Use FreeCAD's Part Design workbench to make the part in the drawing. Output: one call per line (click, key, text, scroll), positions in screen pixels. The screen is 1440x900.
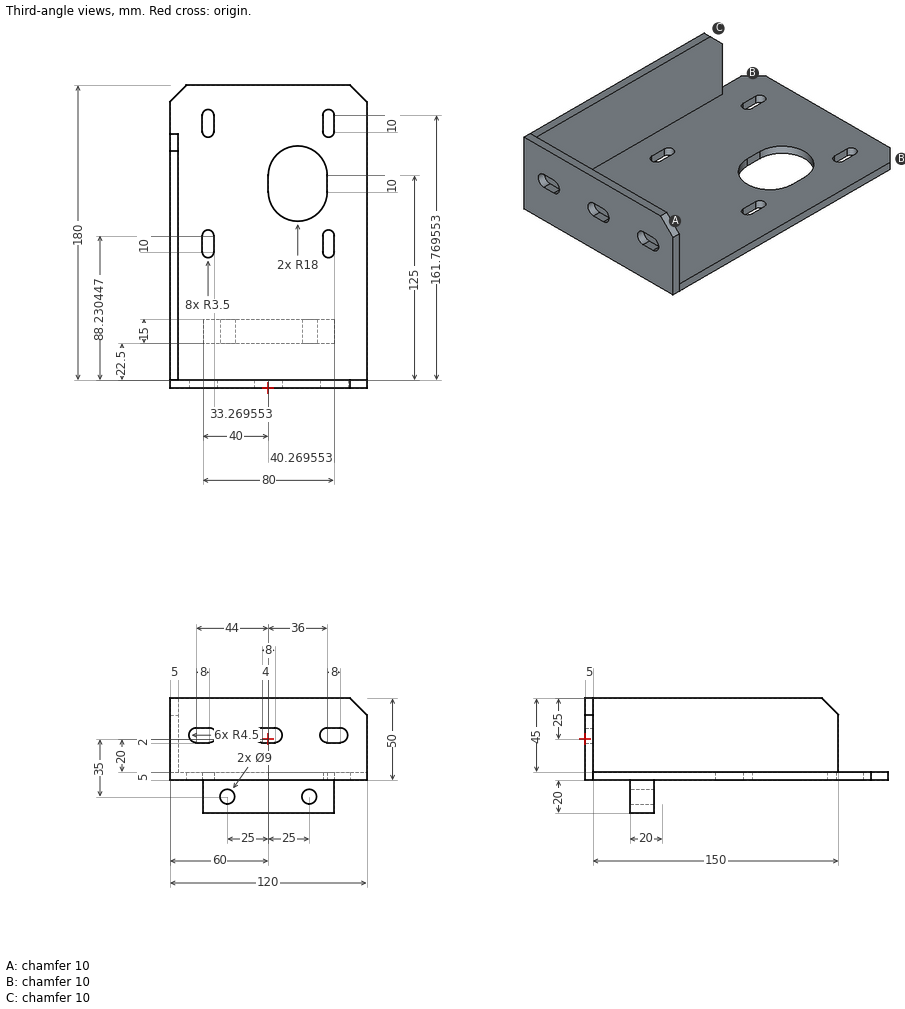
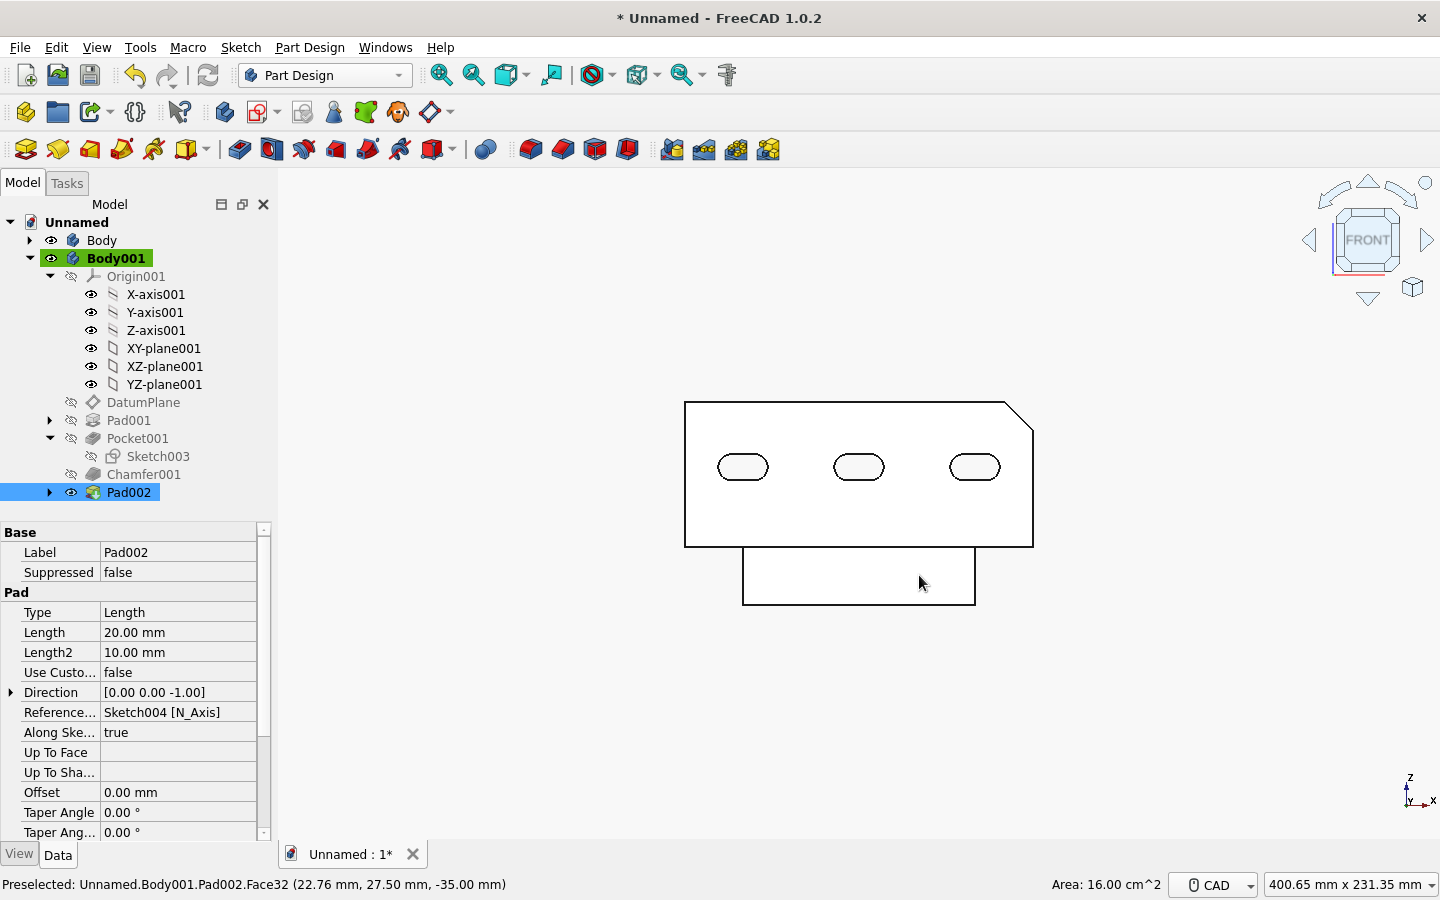
click(258, 112)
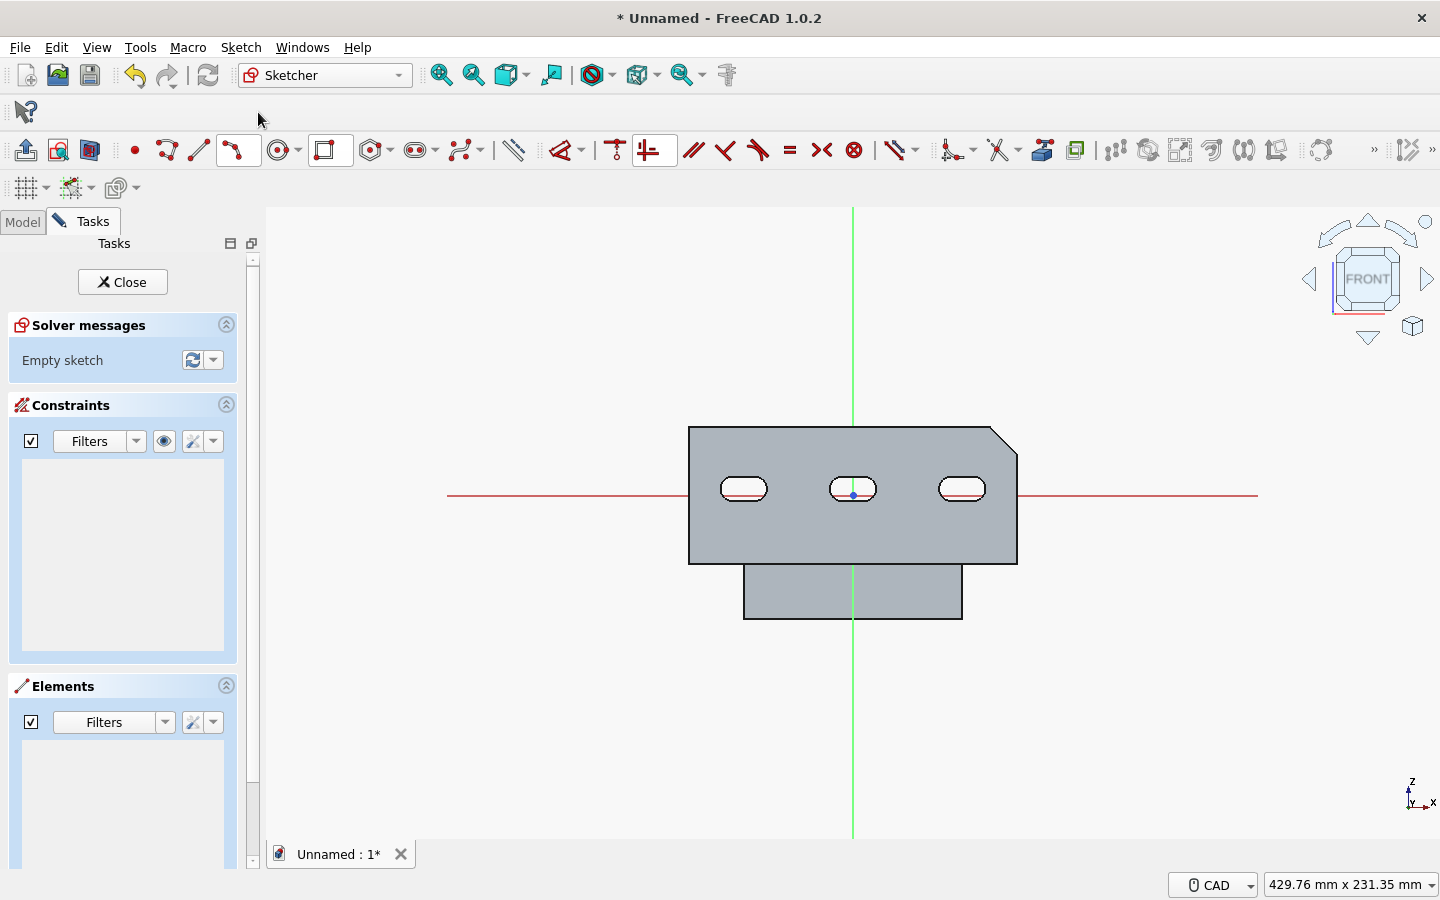
scroll(875, 558, up, 7)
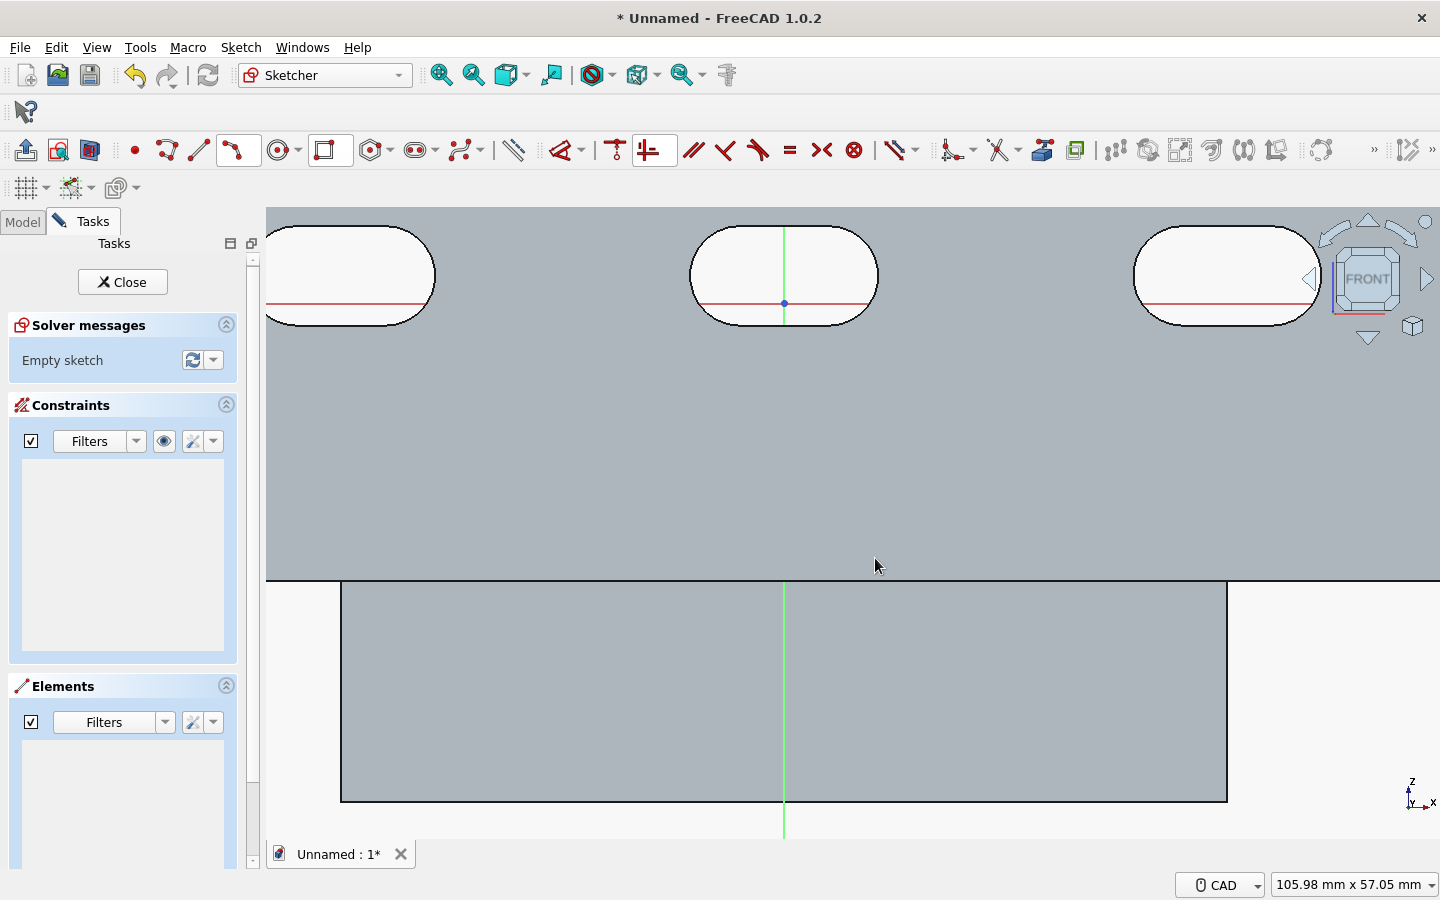
key(g)
key(c)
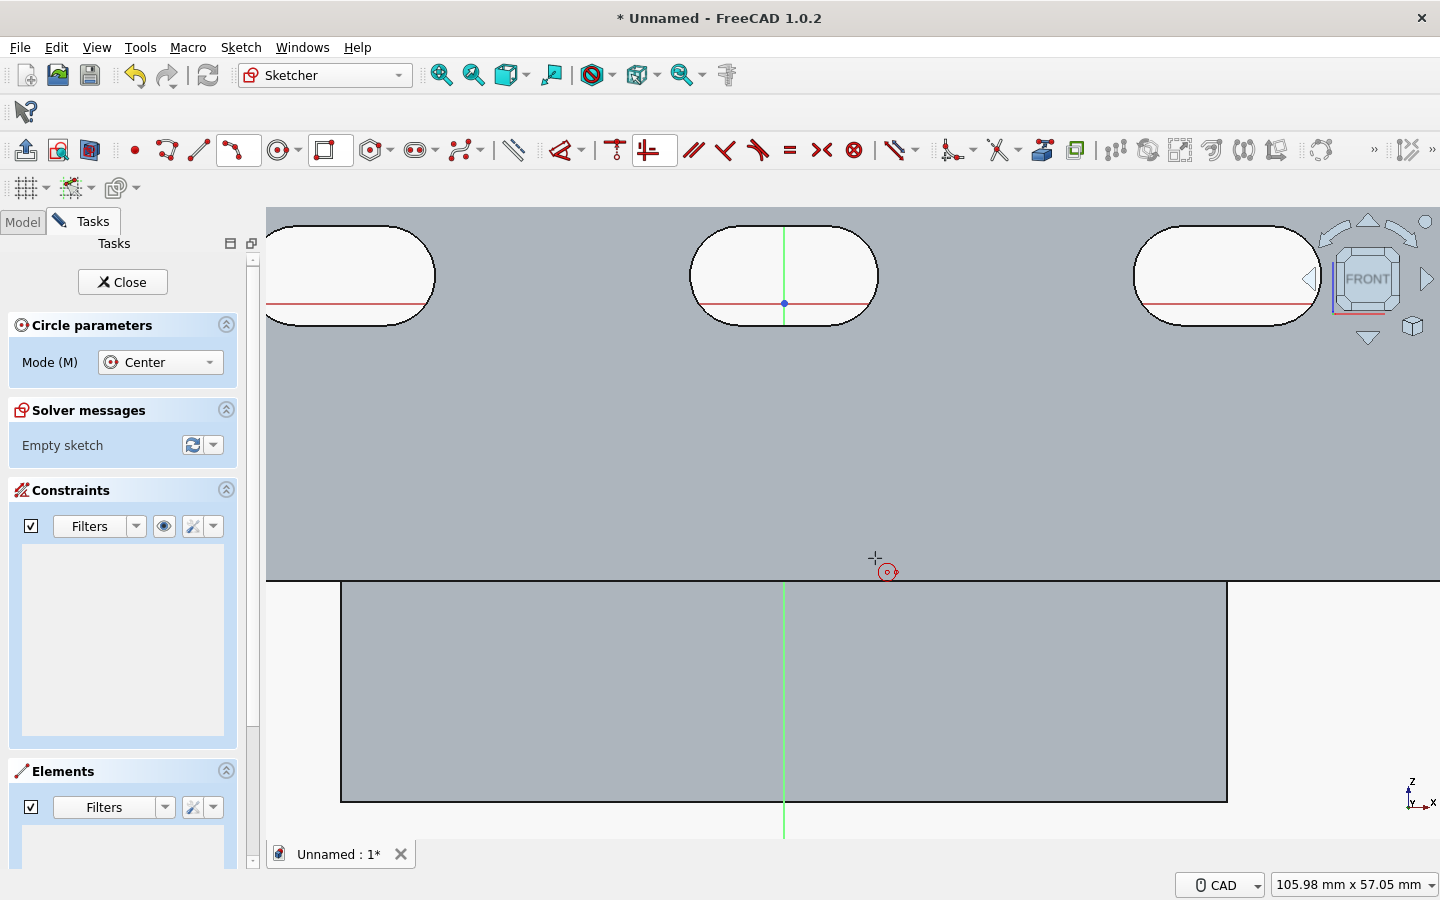
click(507, 691)
click(543, 656)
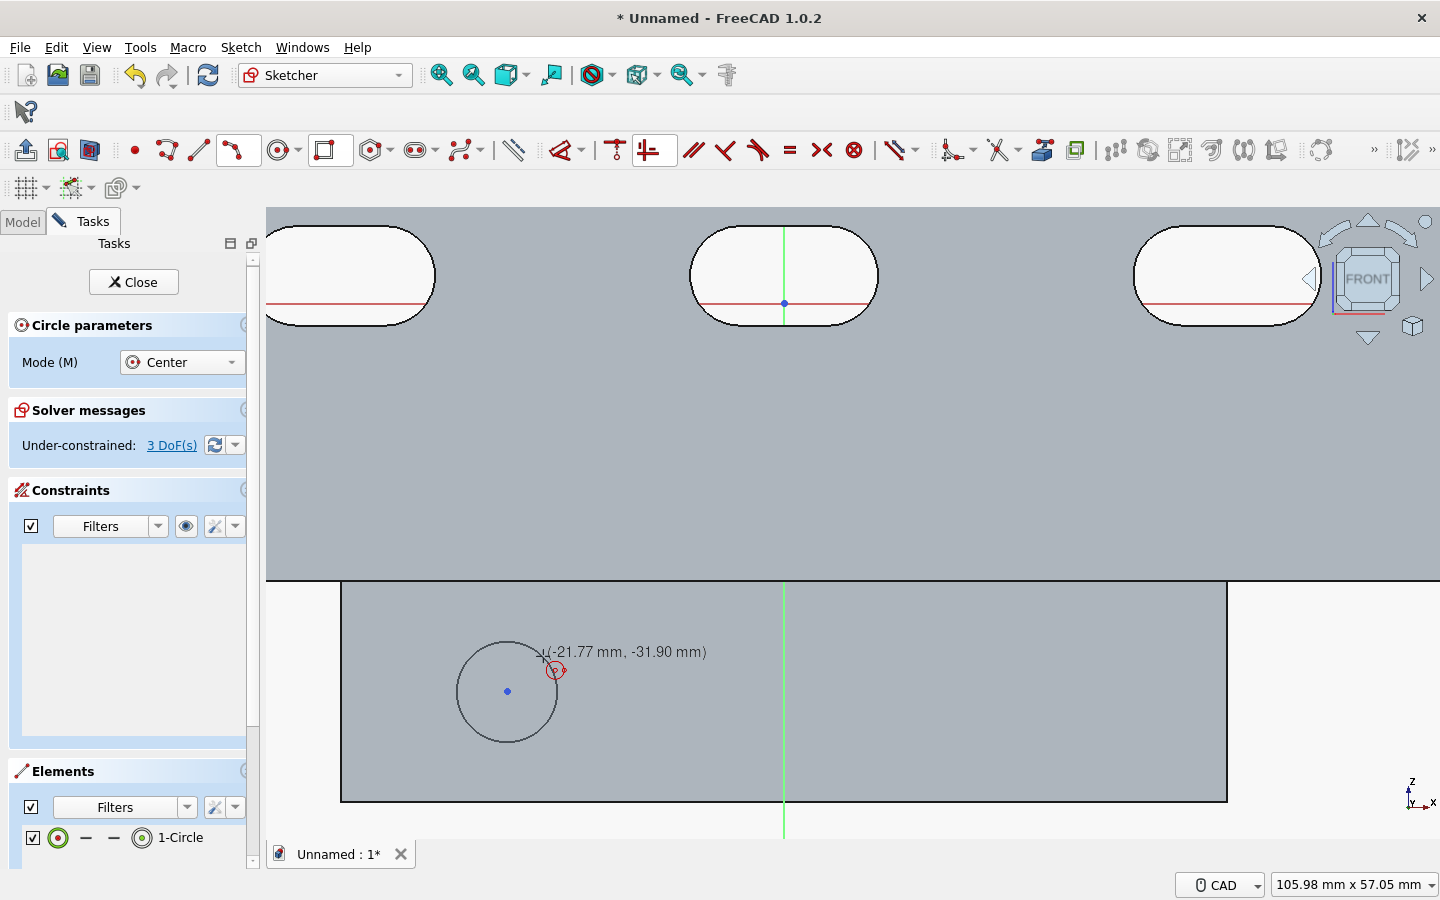
click(1061, 691)
click(1096, 656)
key(Escape)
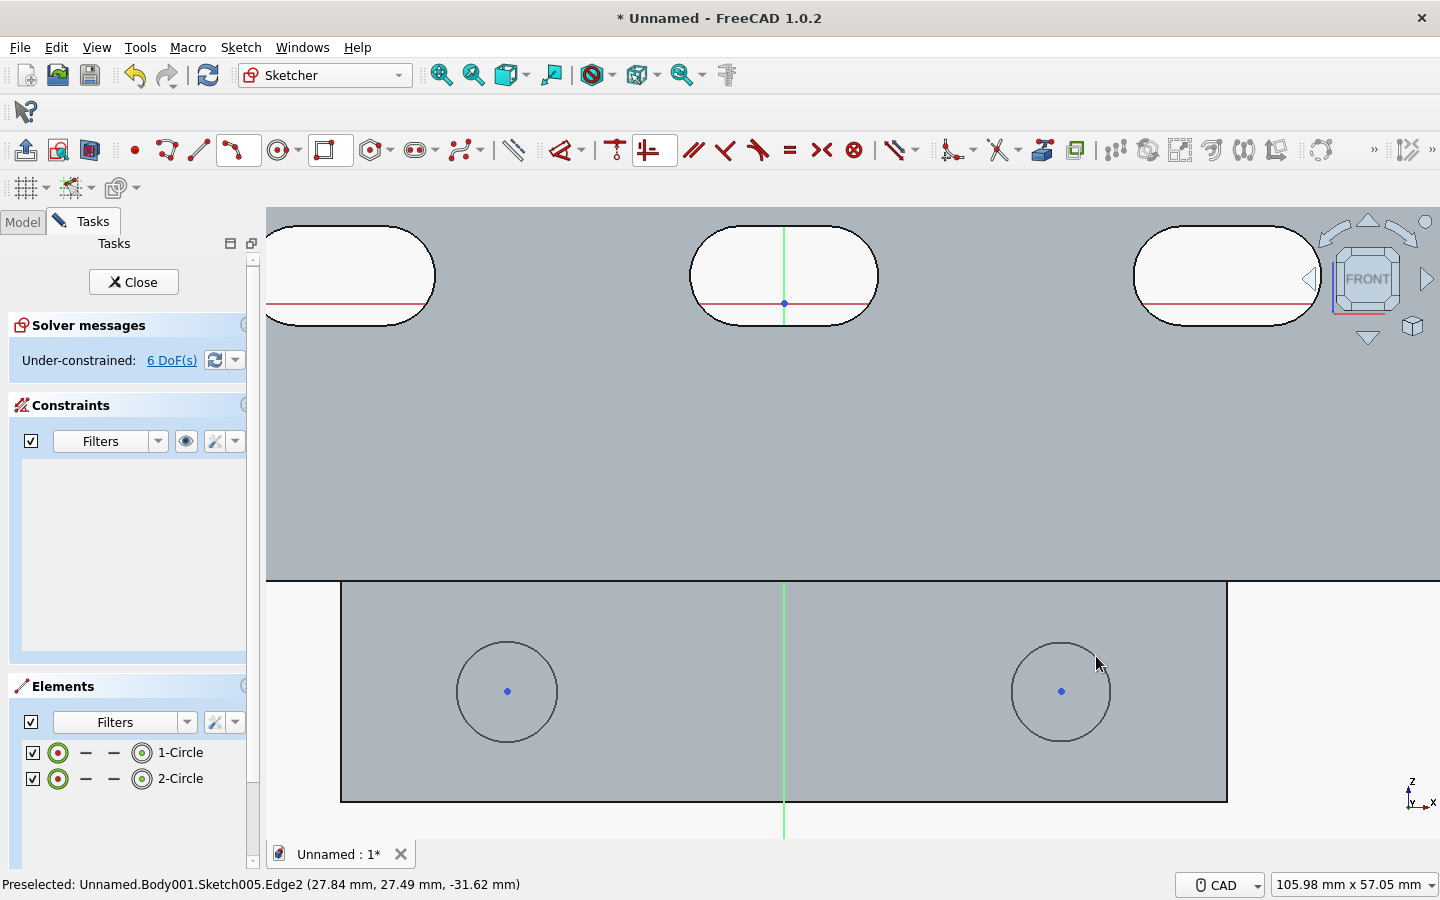
click(542, 656)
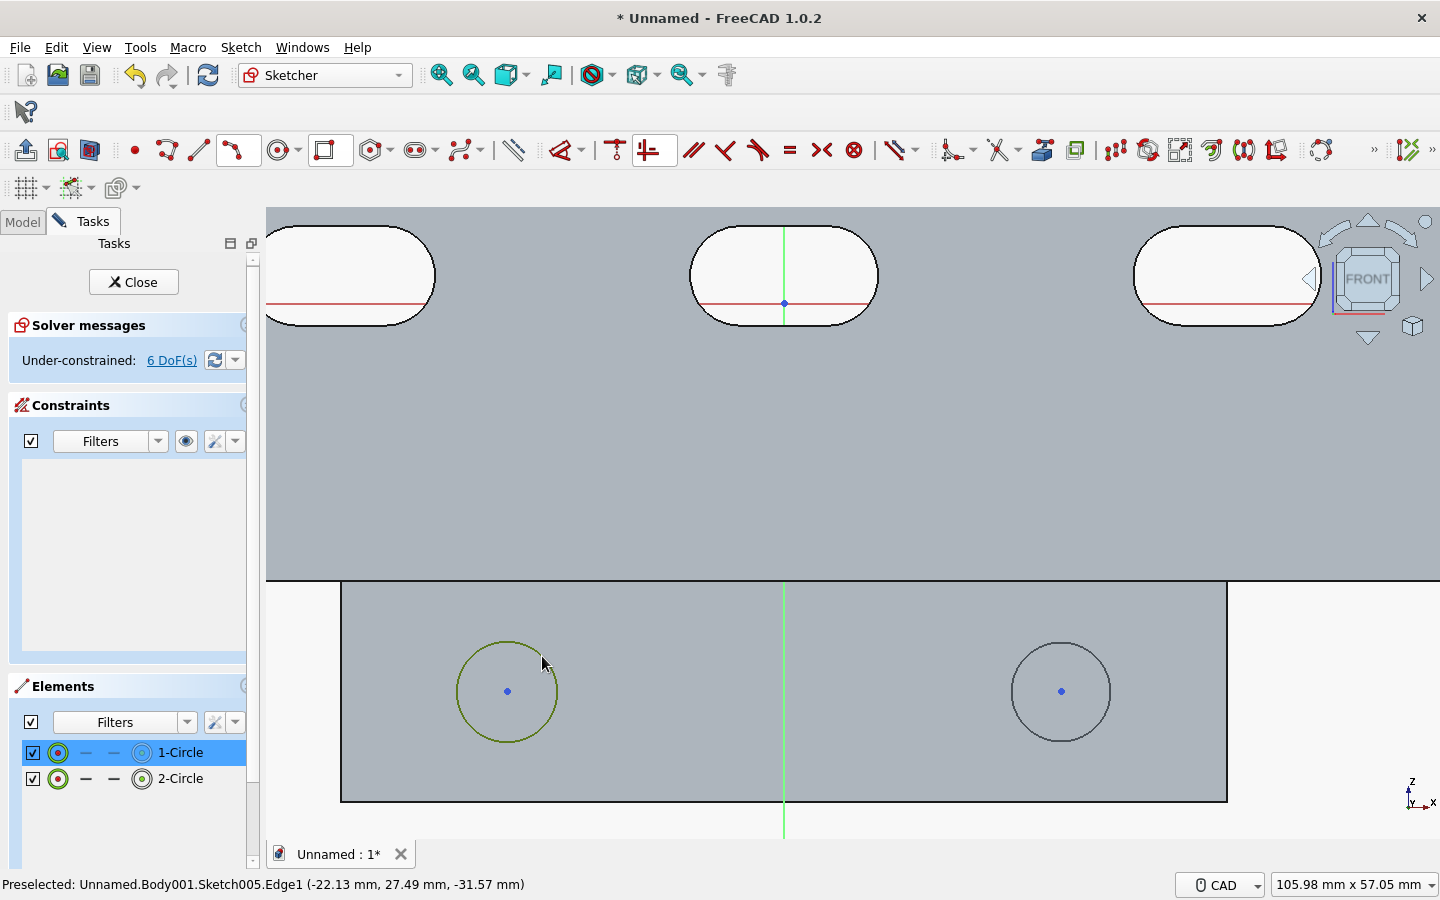
click(1096, 657)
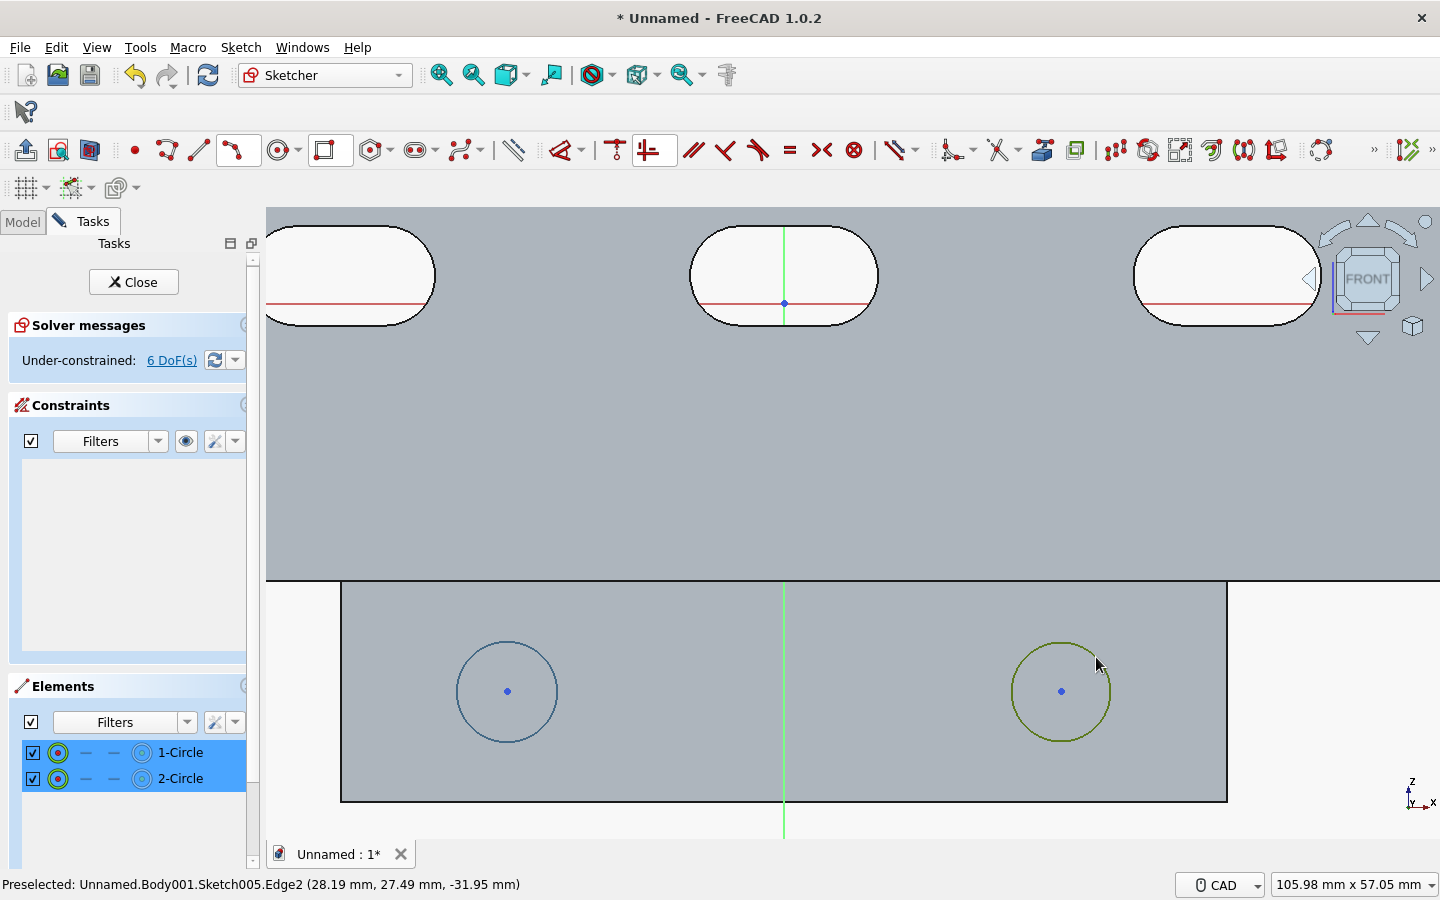
key(e)